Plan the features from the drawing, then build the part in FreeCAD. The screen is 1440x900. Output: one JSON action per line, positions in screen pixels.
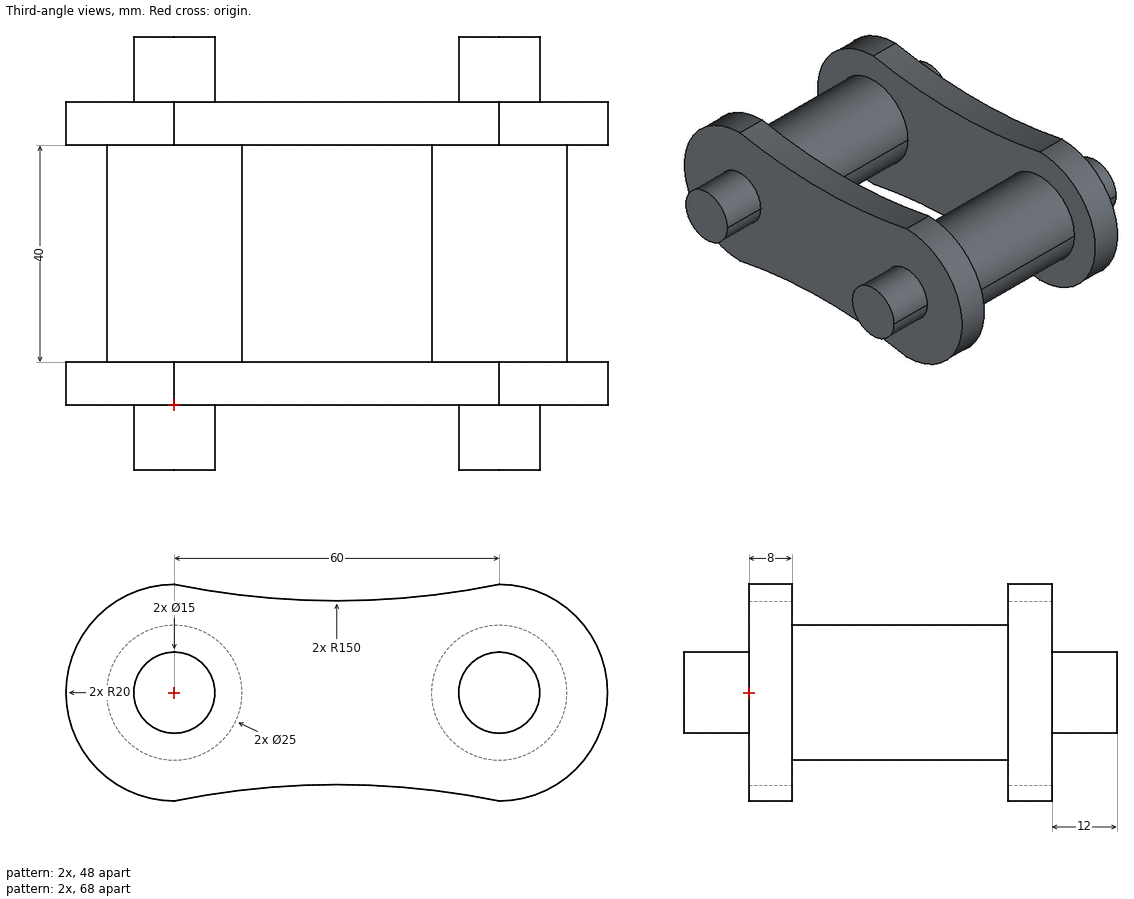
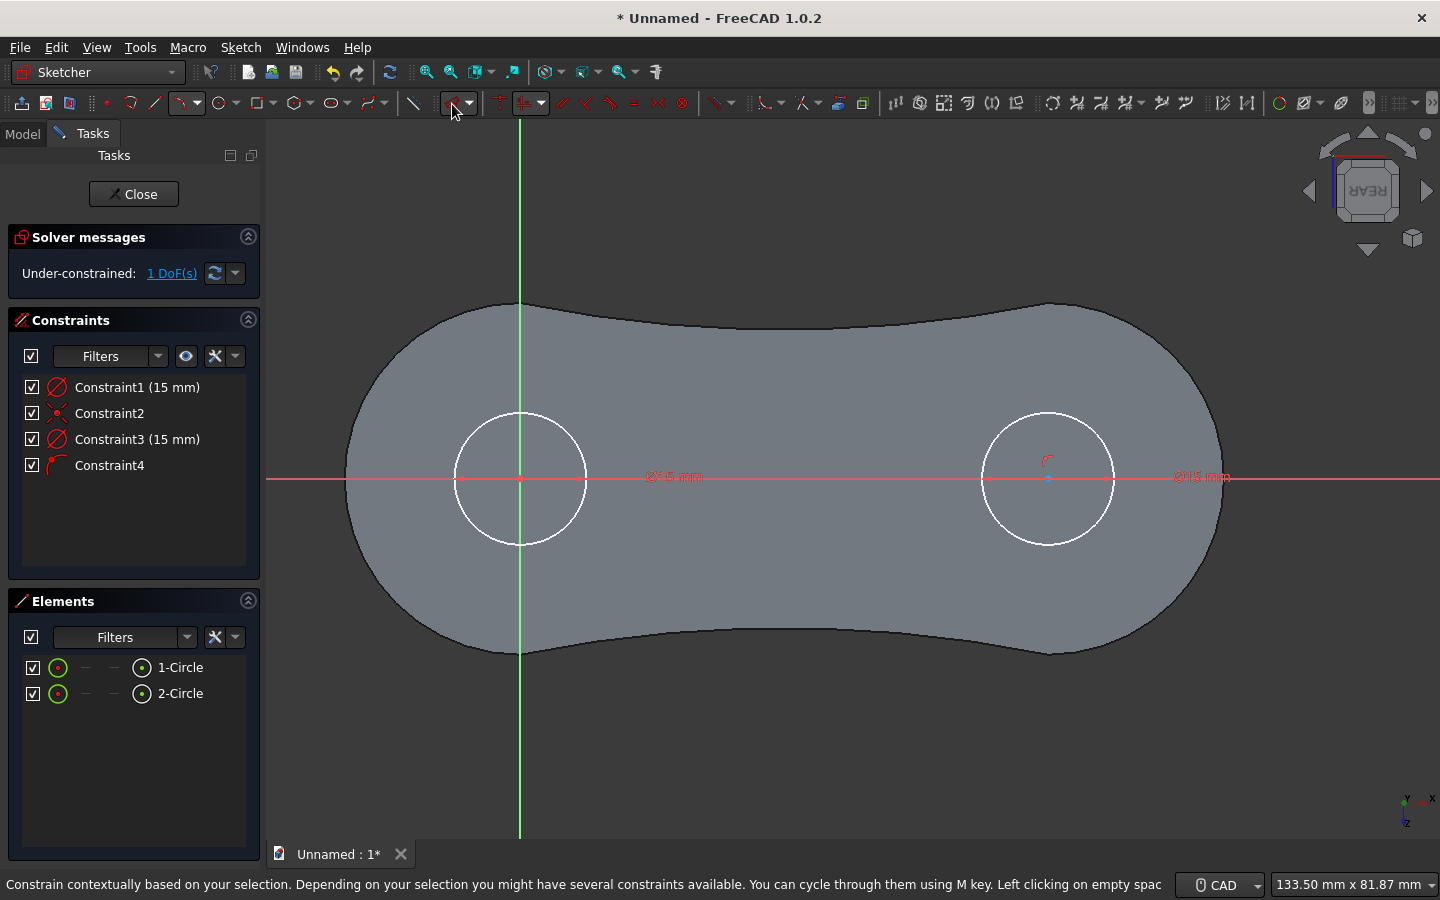
{"action": "left_click", "coordinate": [1048, 479]}
{"action": "left_click", "coordinate": [784, 513]}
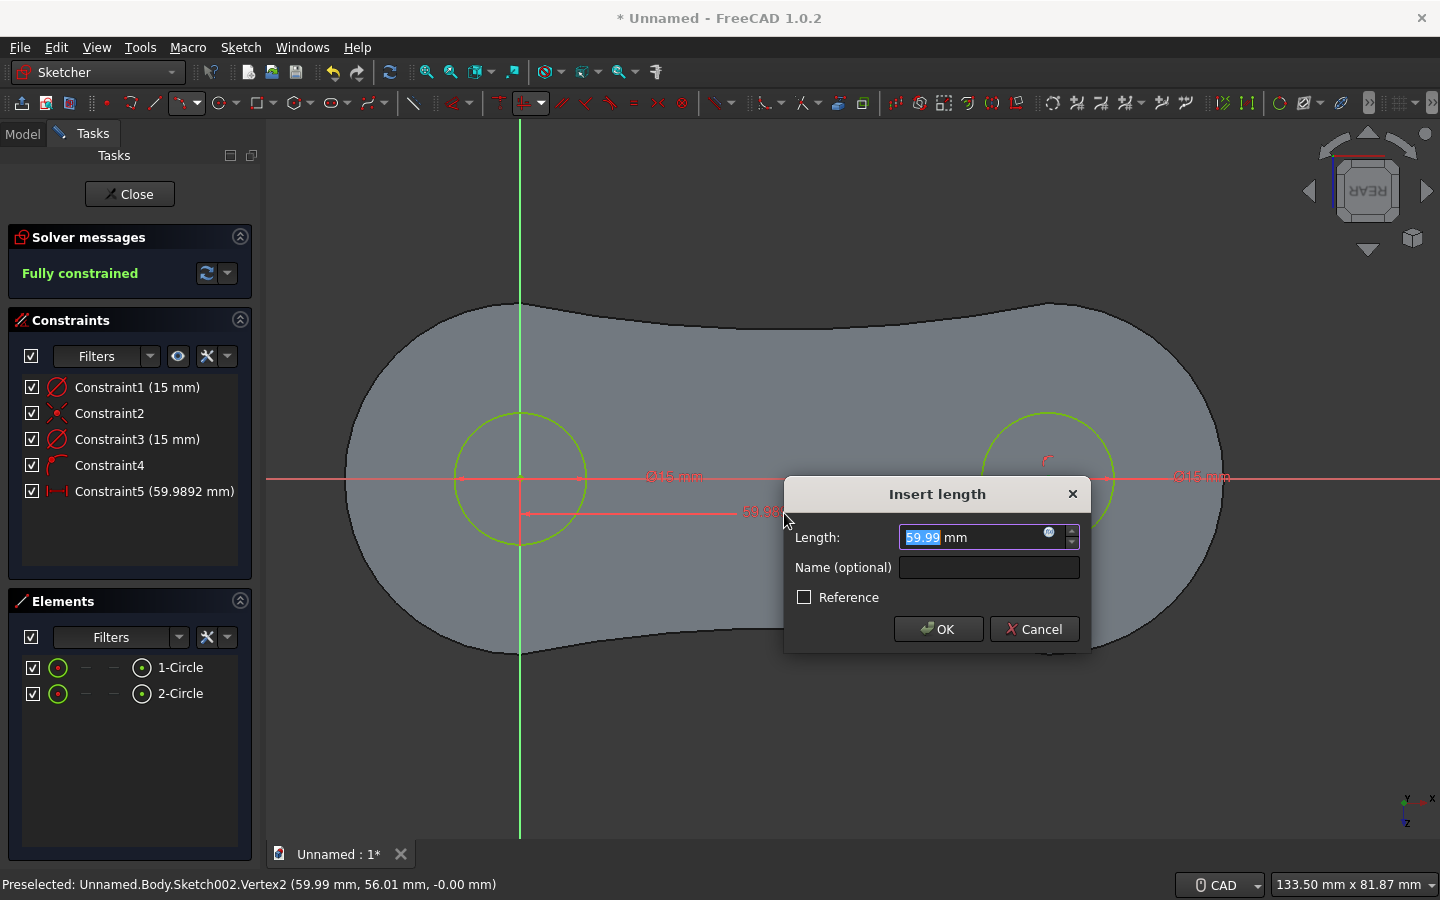
{"action": "type", "text": "60"}
{"action": "key", "text": "Return"}
{"action": "key", "text": "Escape"}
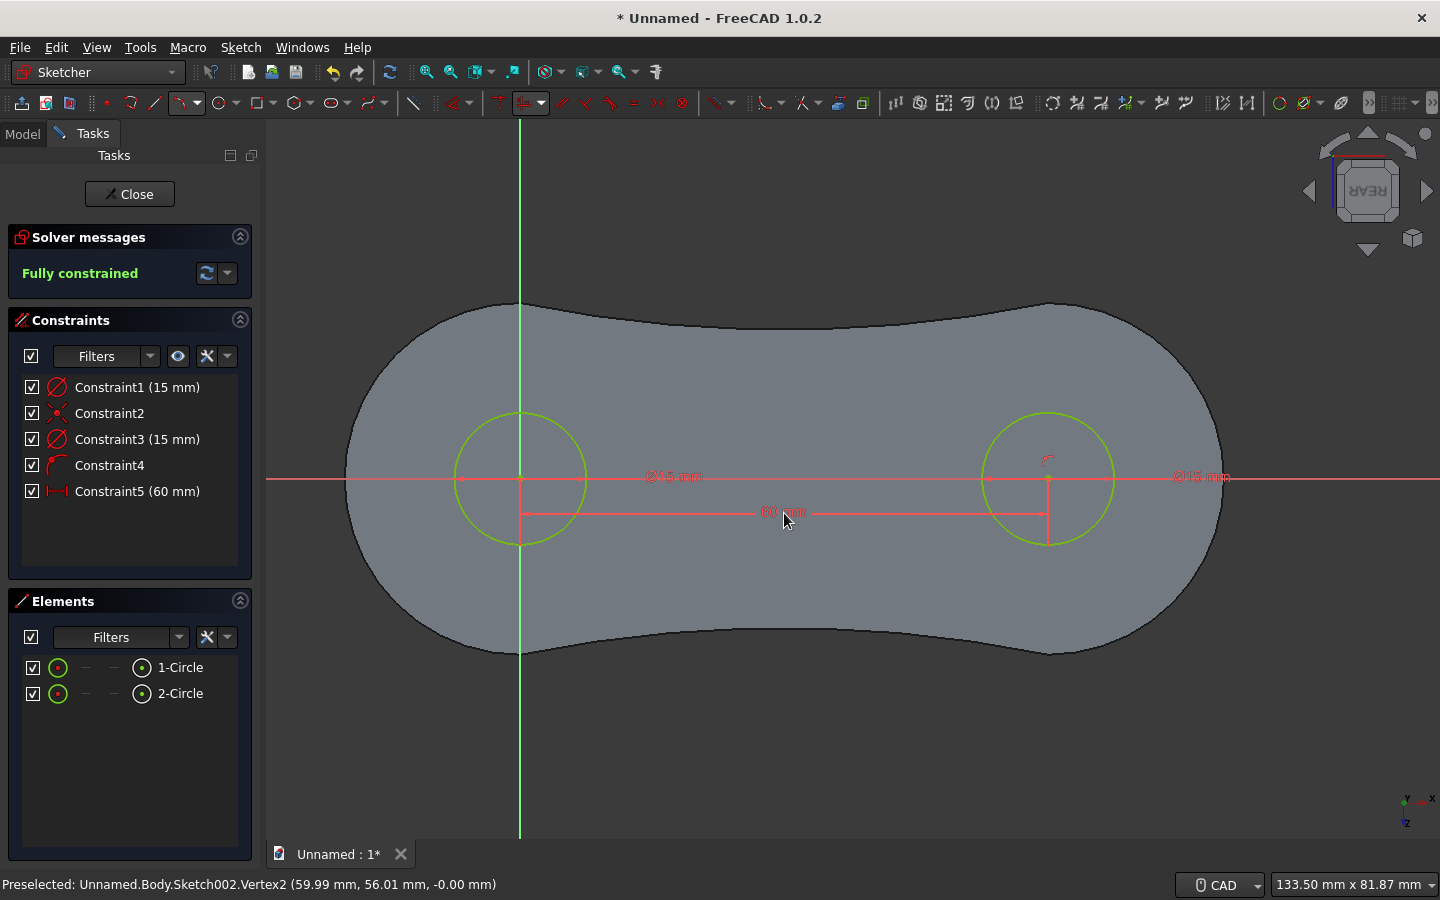
{"action": "left_click", "coordinate": [130, 194]}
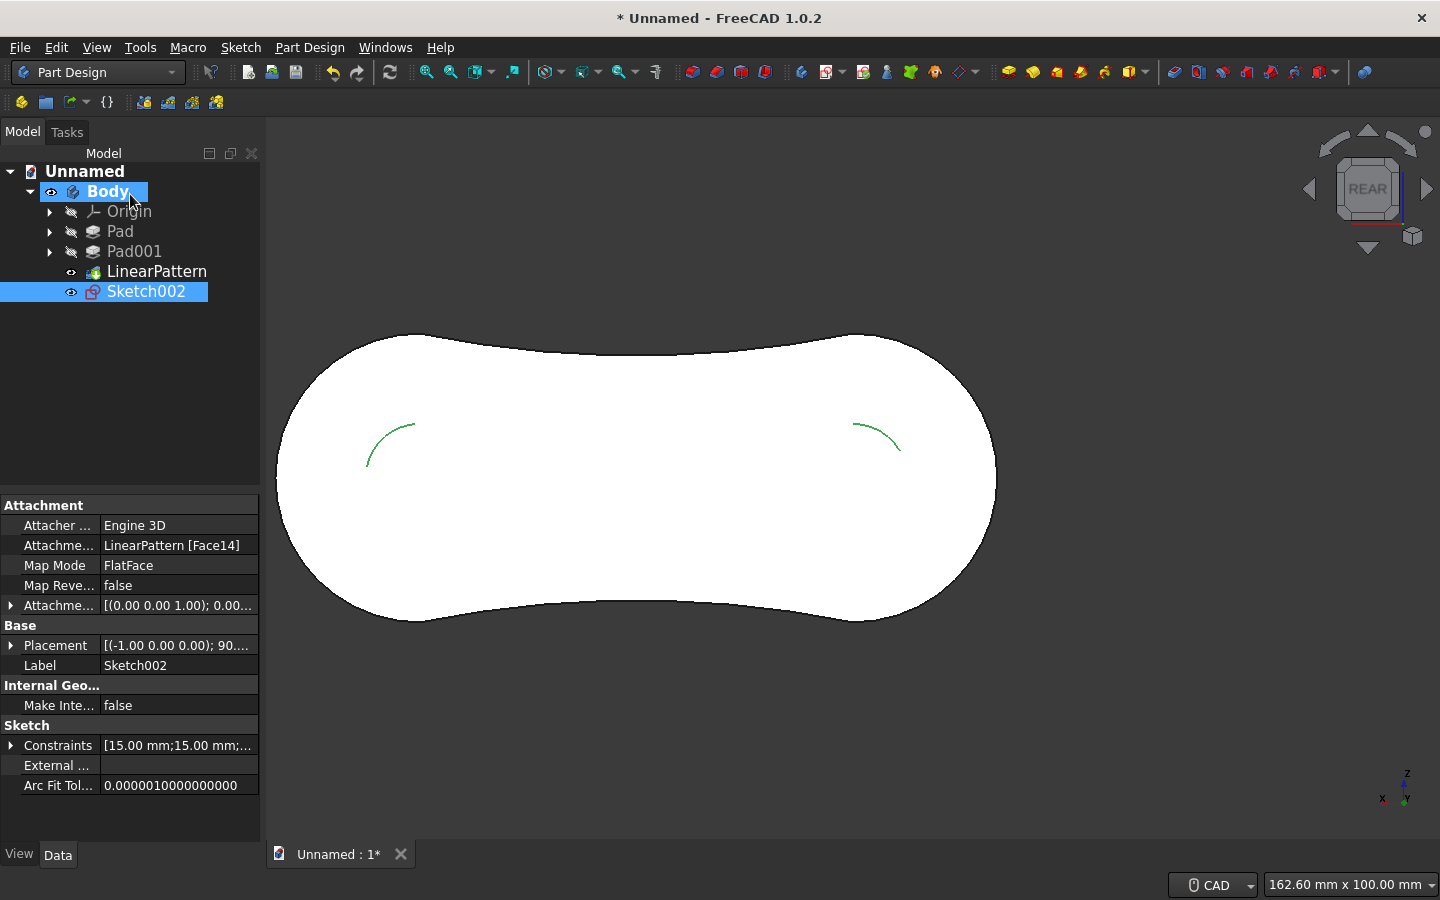
{"action": "left_click", "coordinate": [1010, 72]}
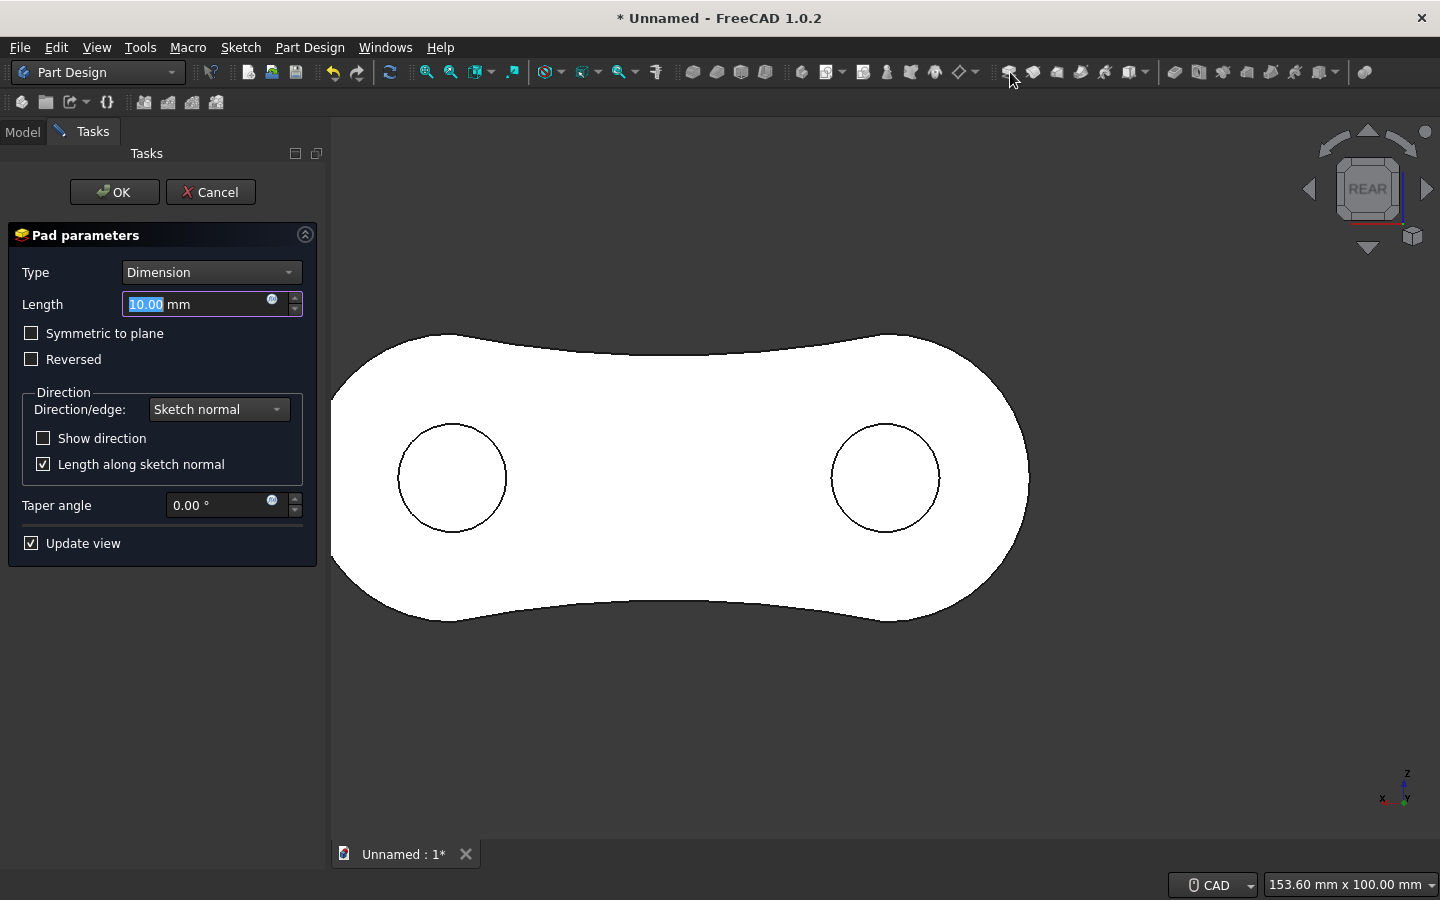
{"action": "type", "text": "12"}
{"action": "key", "text": "Tab"}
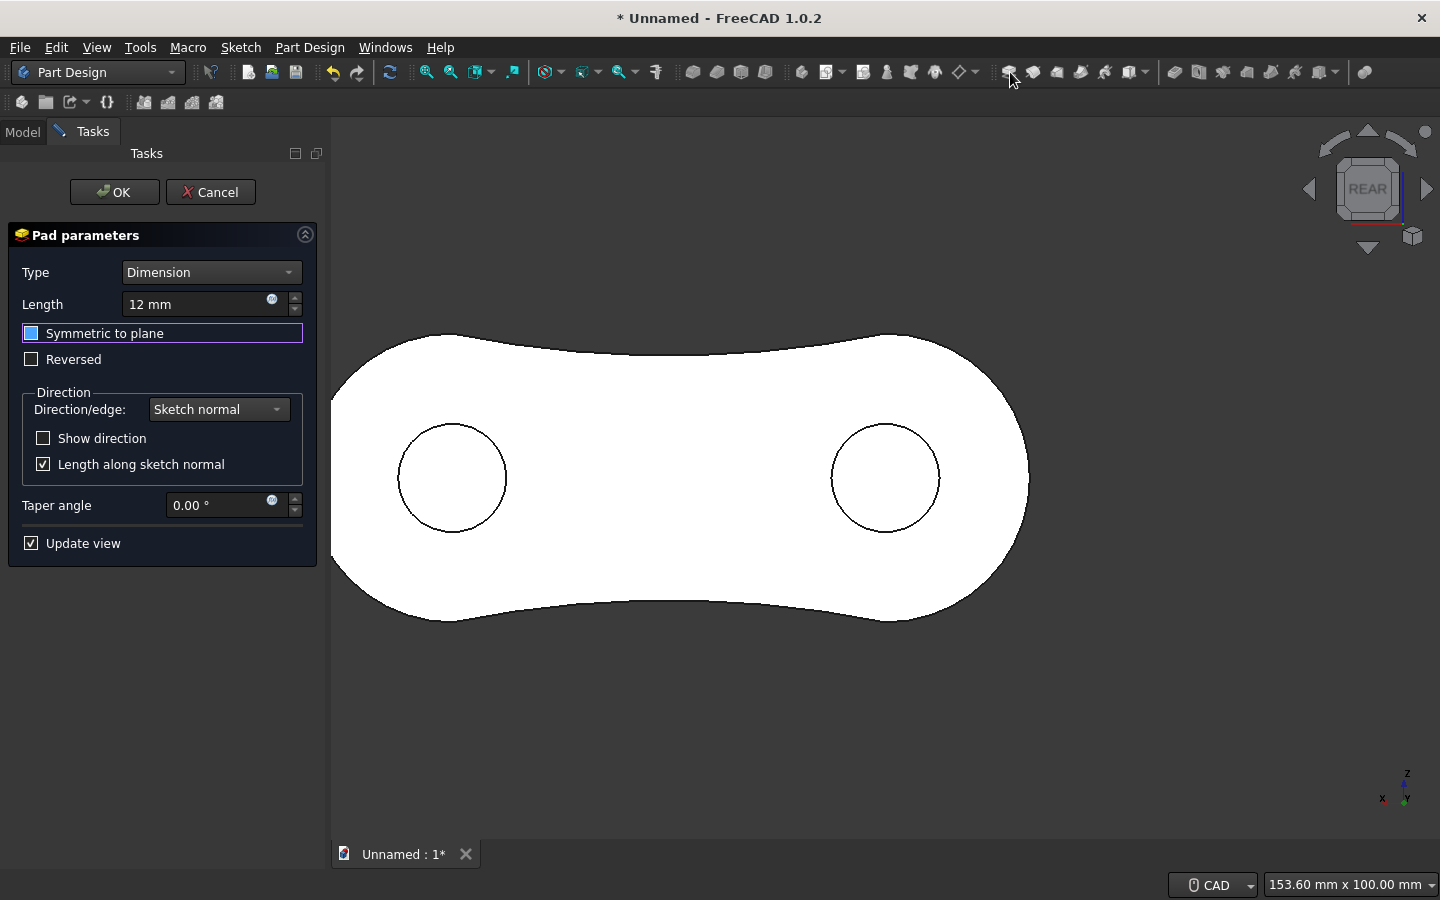
{"action": "left_click", "coordinate": [115, 192]}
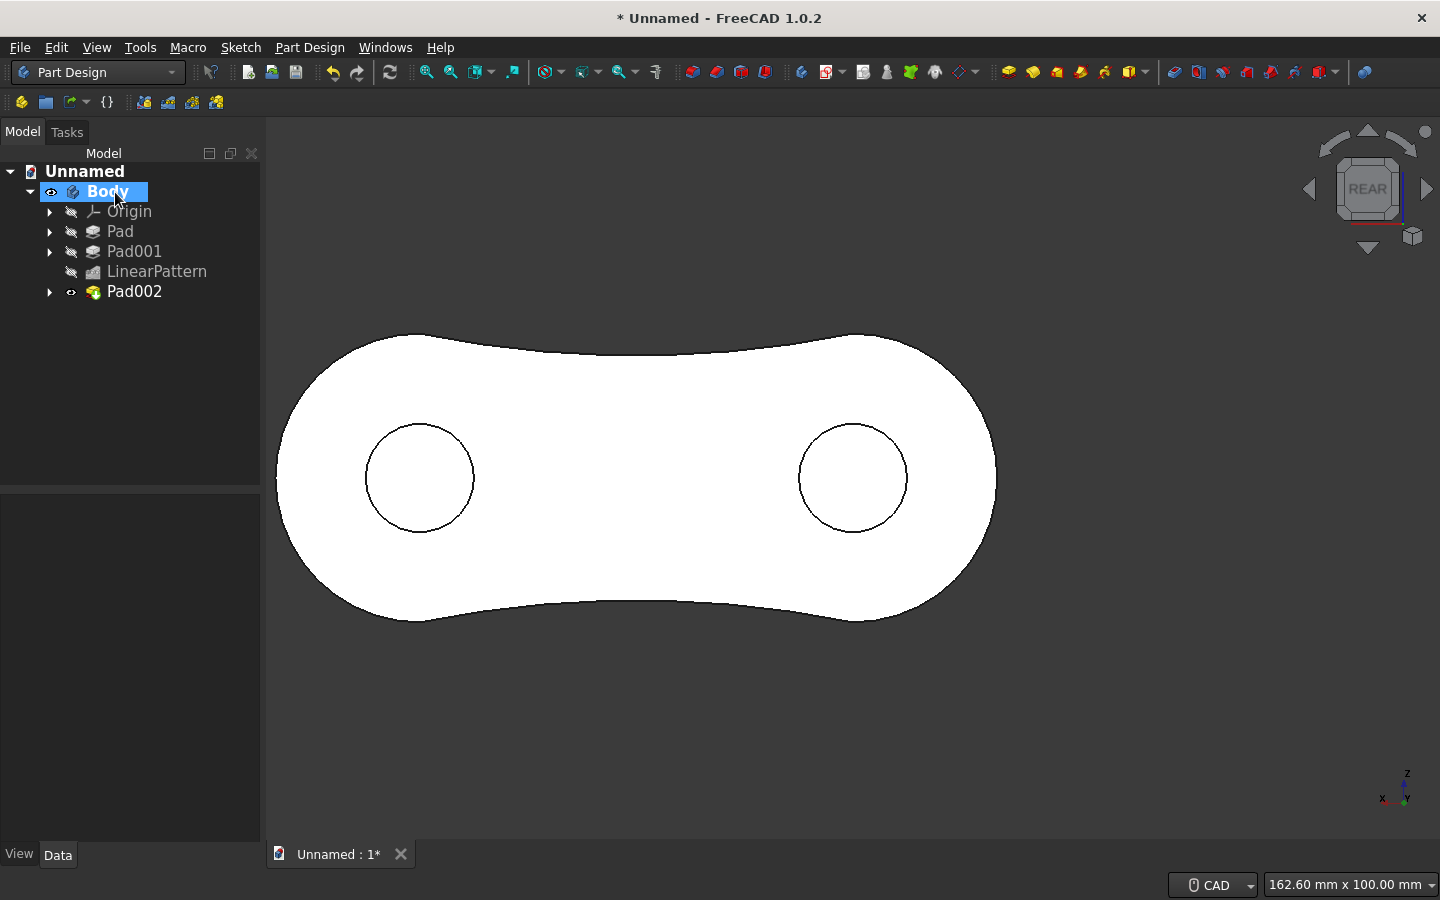
{"action": "left_click", "coordinate": [116, 292]}